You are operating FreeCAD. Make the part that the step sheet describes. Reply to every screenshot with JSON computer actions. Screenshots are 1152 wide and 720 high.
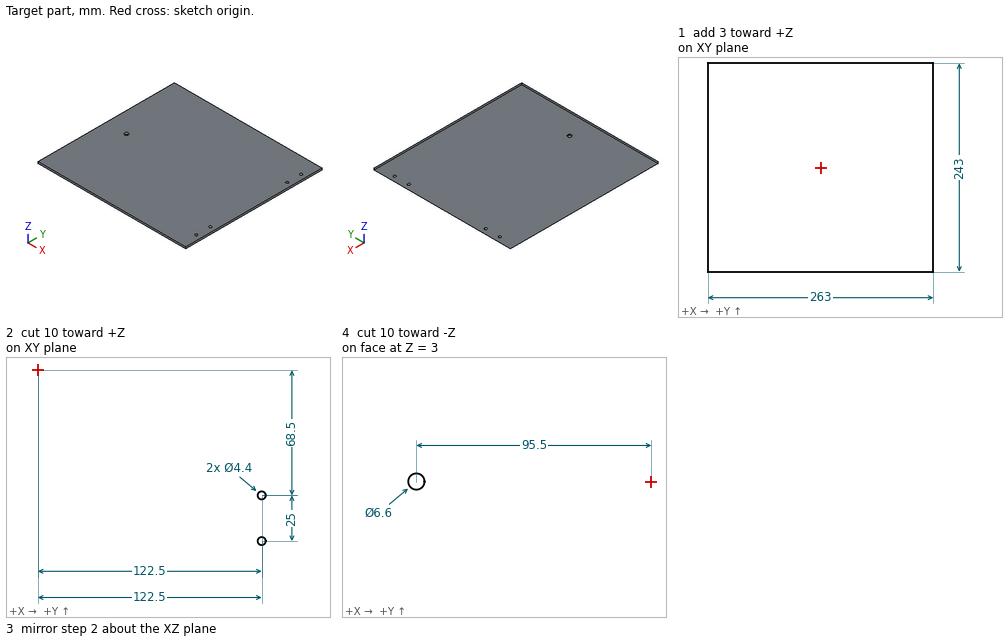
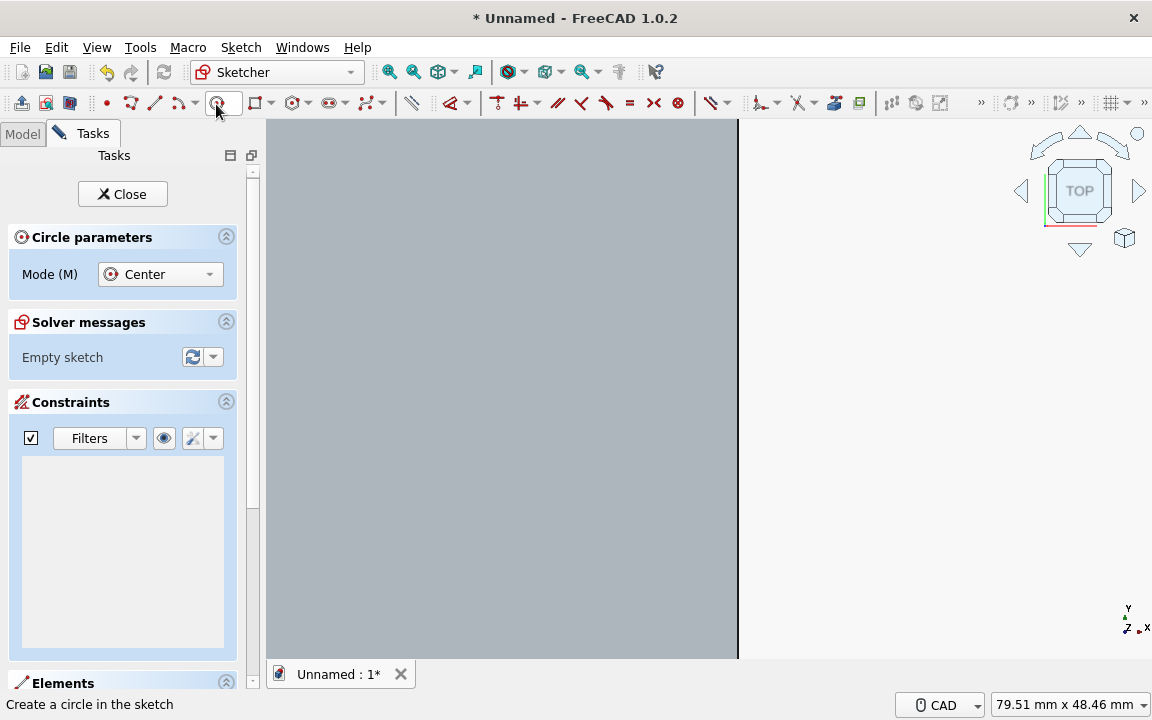
{"action": "left_click", "coordinate": [638, 247]}
{"action": "left_click", "coordinate": [655, 229]}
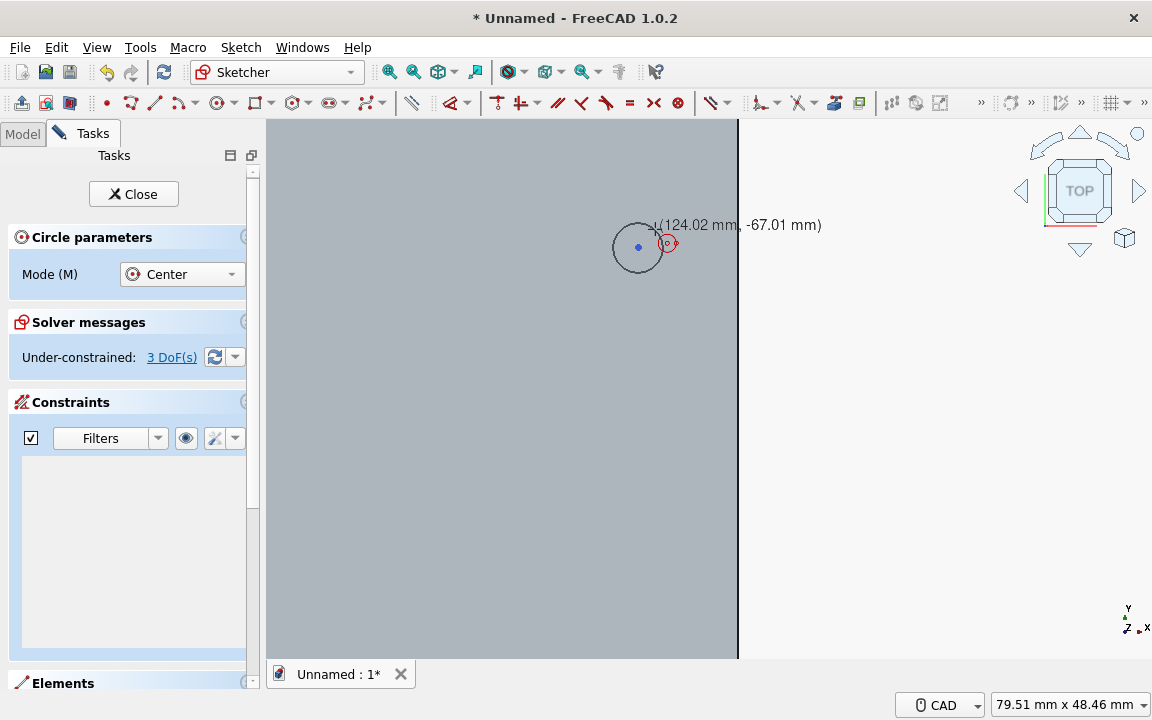
{"action": "left_click", "coordinate": [638, 525]}
{"action": "left_click", "coordinate": [655, 508]}
{"action": "key", "text": "Escape"}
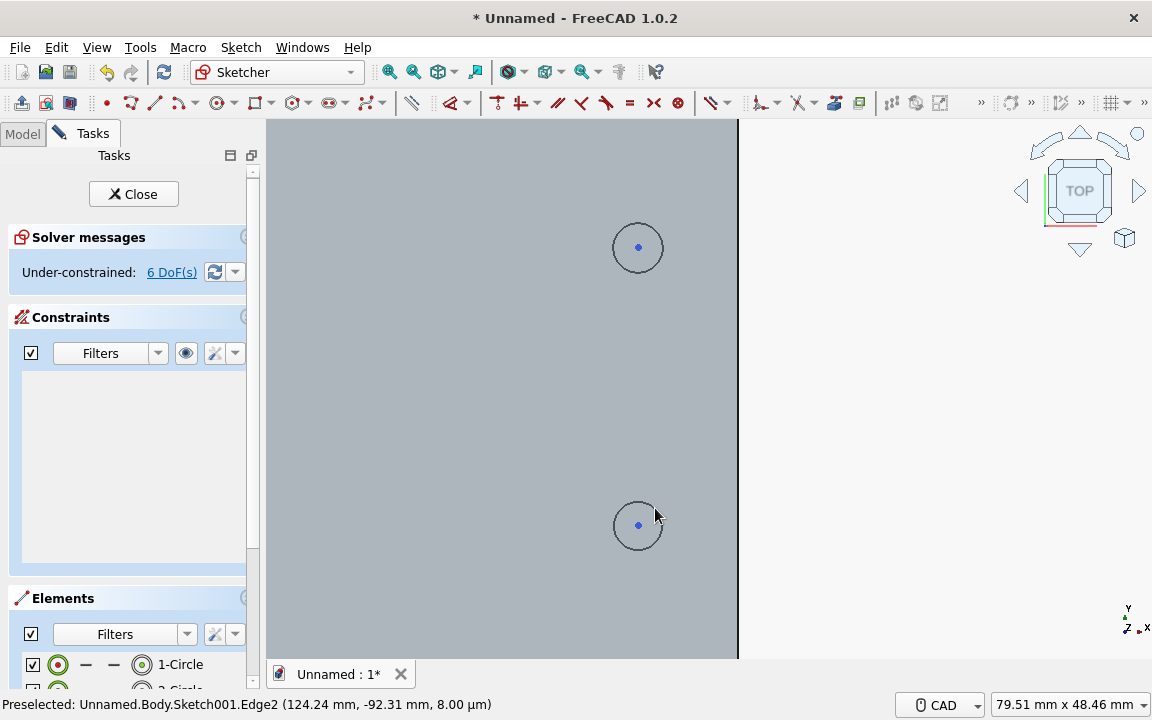
{"action": "left_click", "coordinate": [655, 230]}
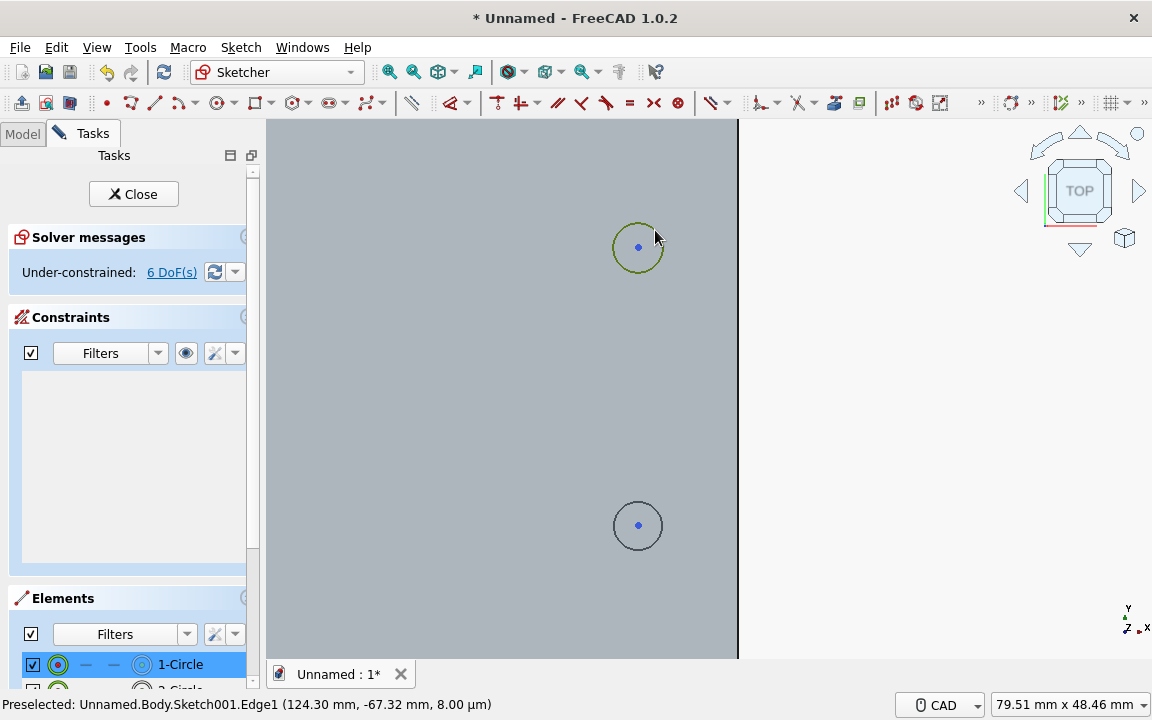
{"action": "left_click", "coordinate": [655, 509]}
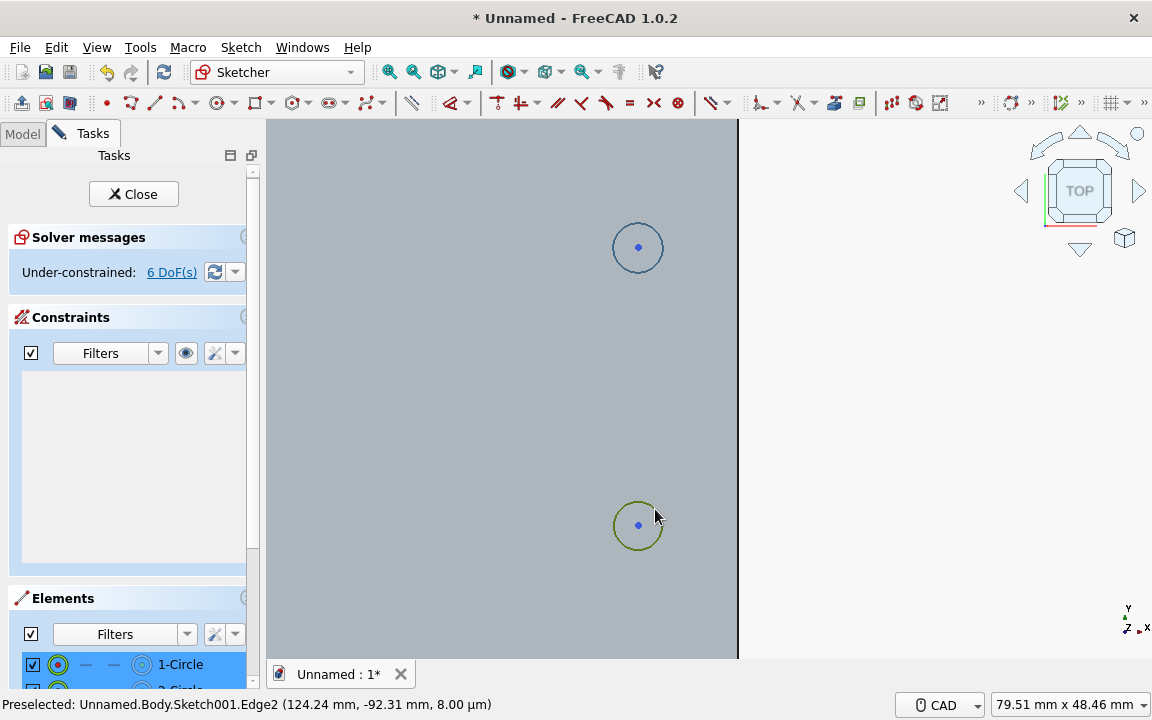
{"action": "key", "text": "e"}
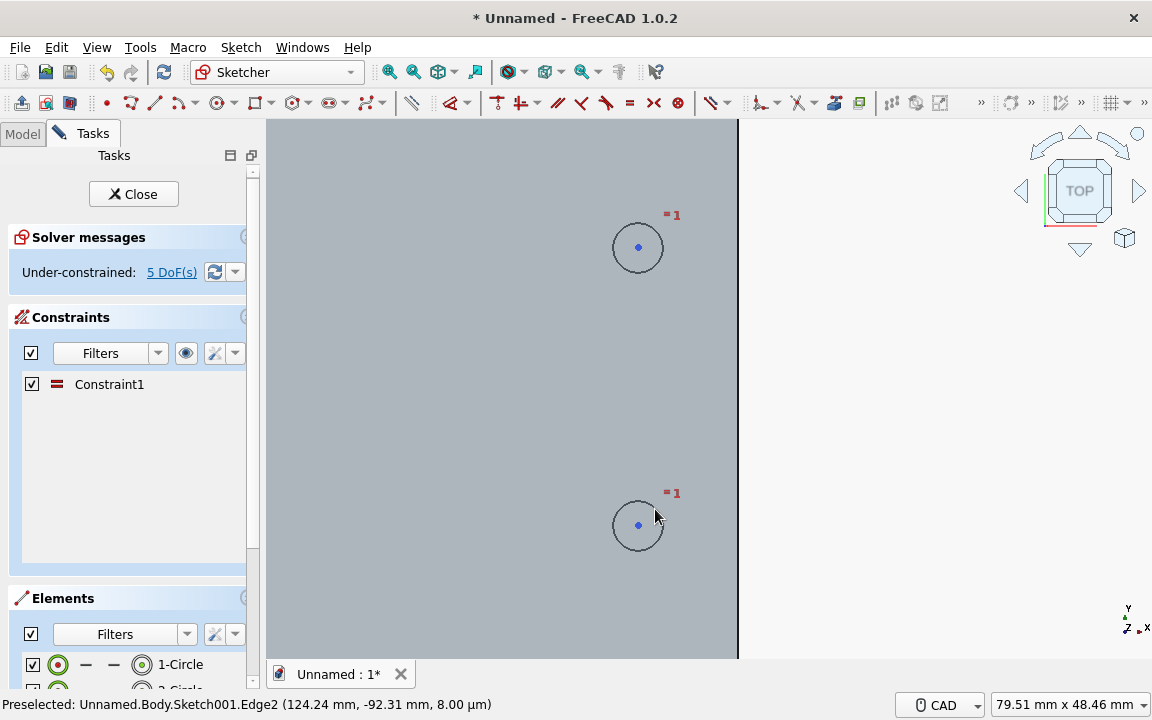
{"action": "left_click", "coordinate": [655, 230]}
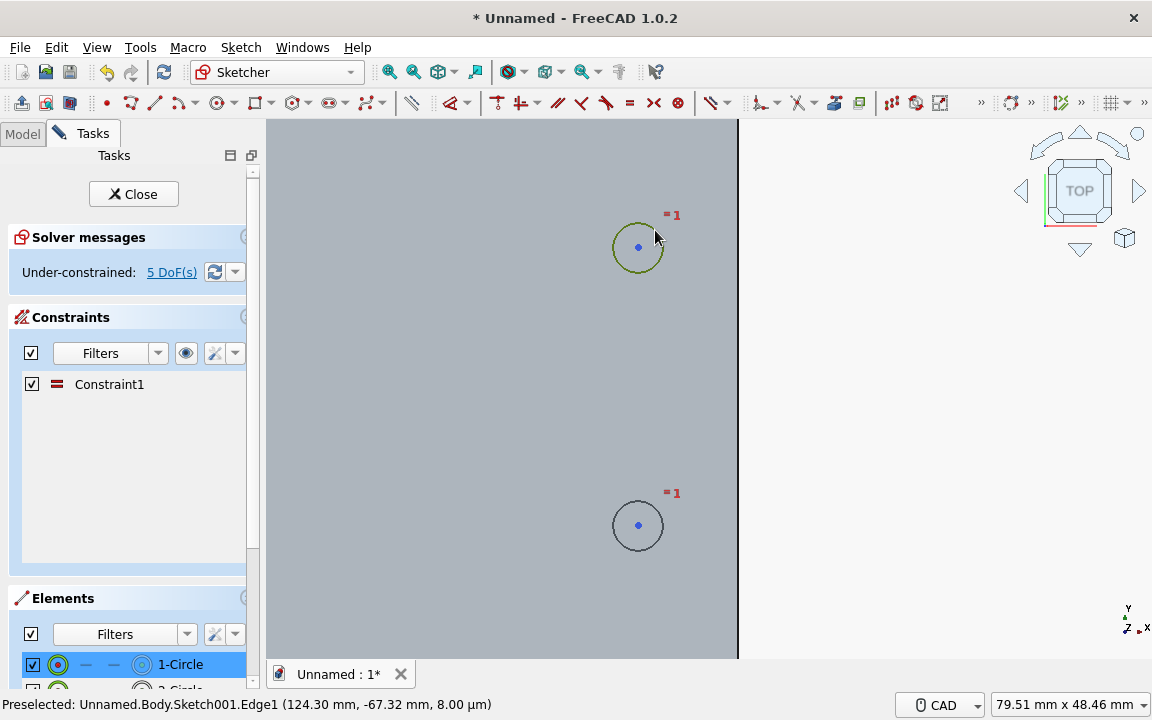
{"action": "key", "text": "k o"}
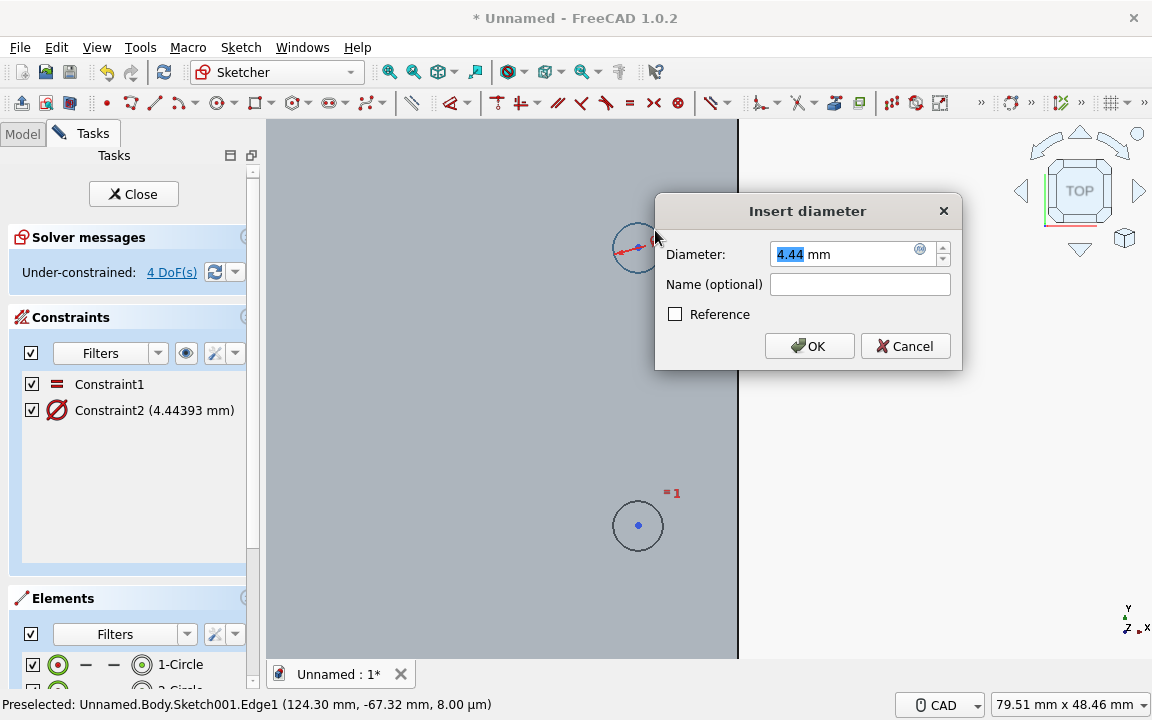
{"action": "type", "text": "4.4"}
{"action": "key", "text": "Return"}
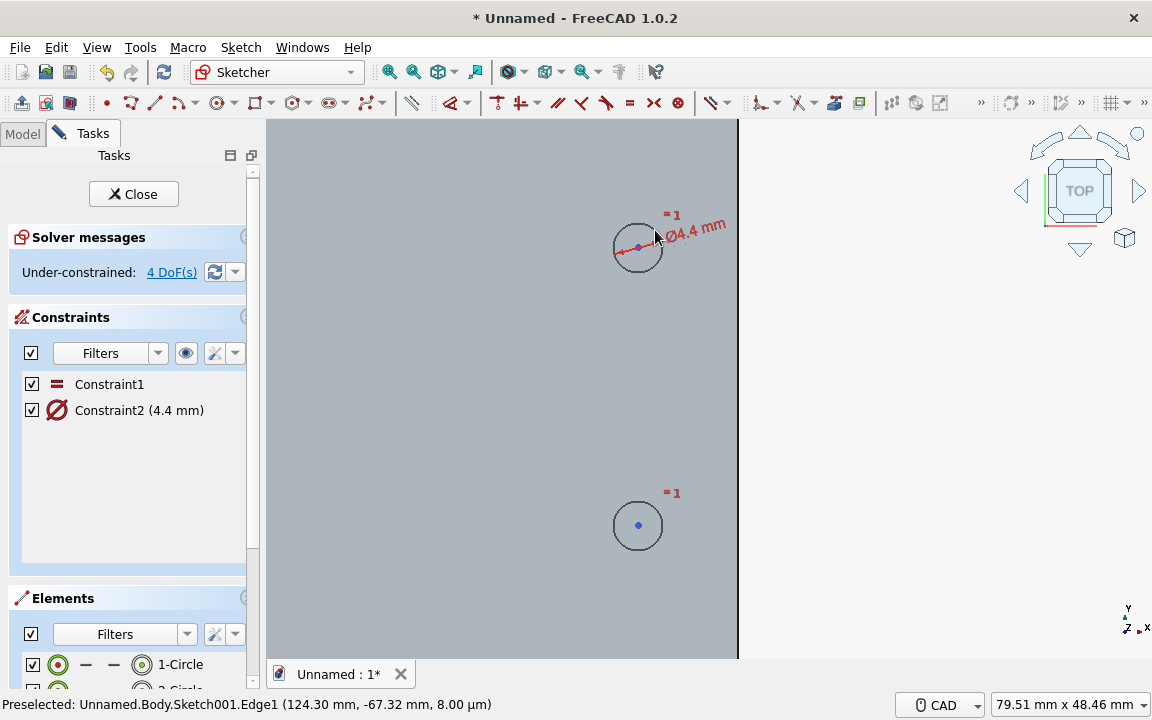
{"action": "left_click", "coordinate": [638, 248]}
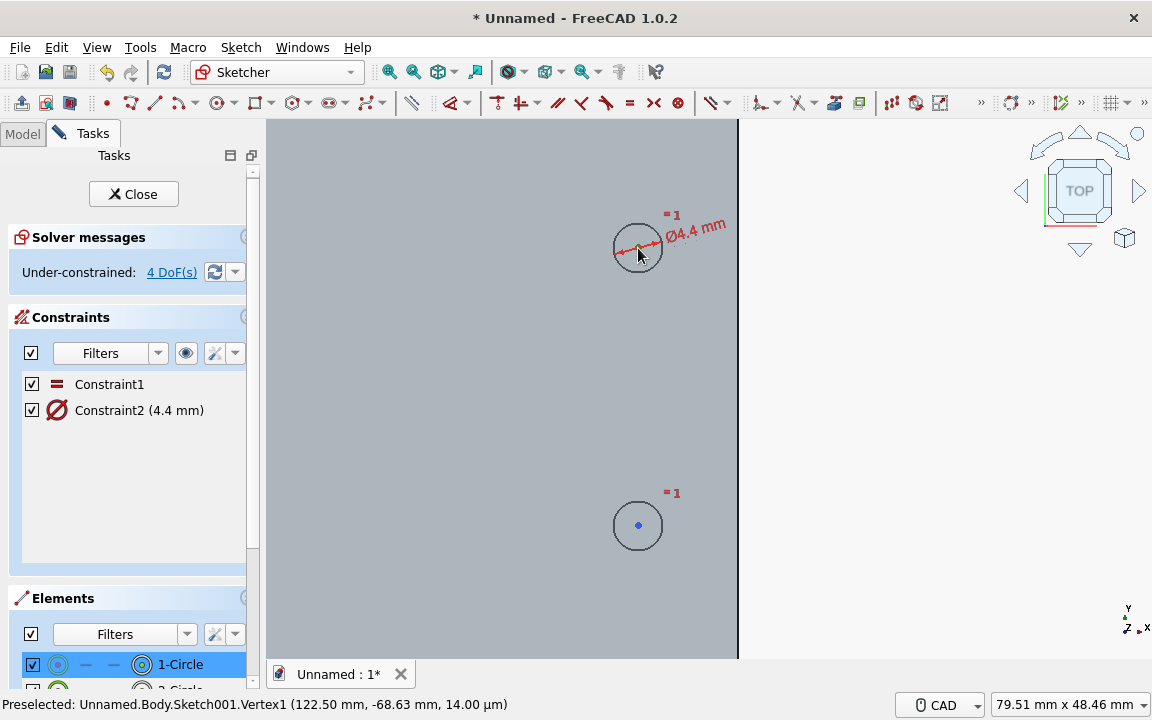
{"action": "left_click", "coordinate": [638, 526]}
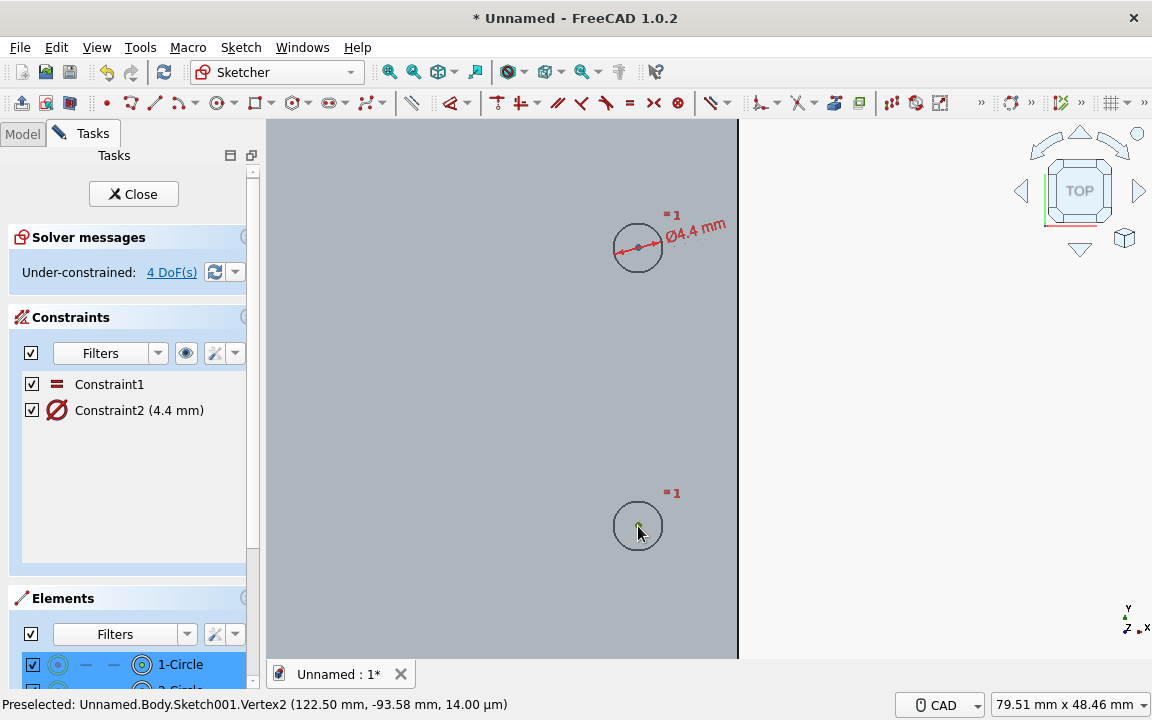
{"action": "key", "text": "i"}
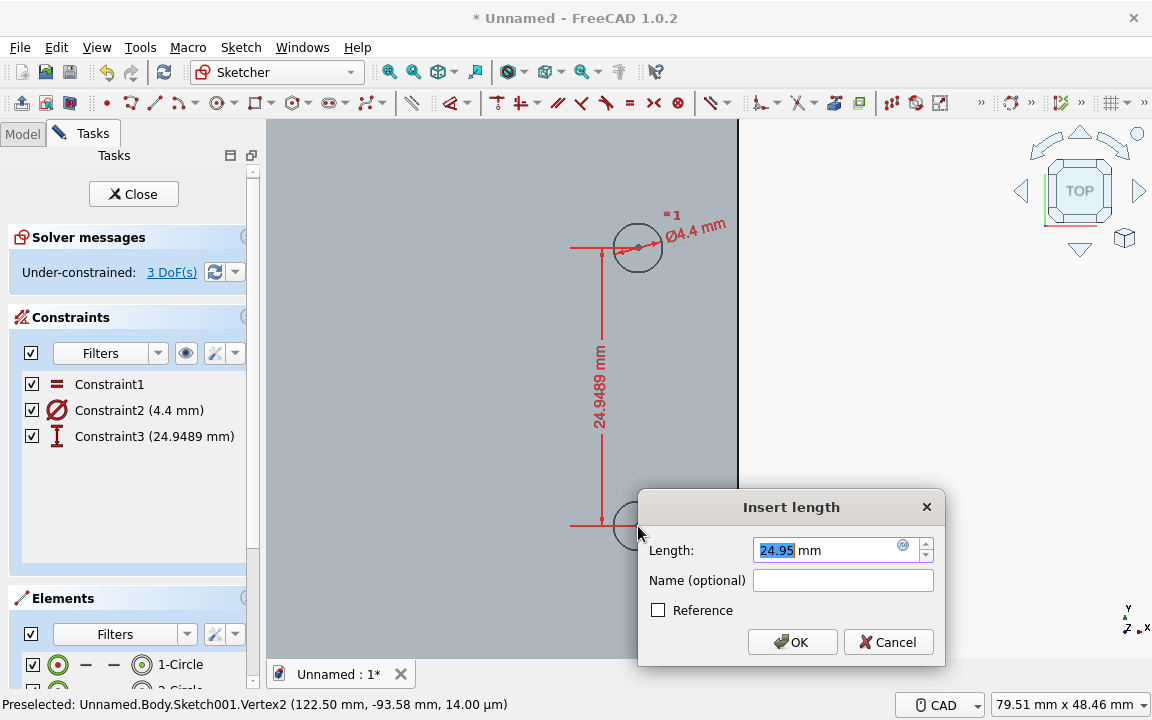
{"action": "type", "text": "25"}
{"action": "key", "text": "Return"}